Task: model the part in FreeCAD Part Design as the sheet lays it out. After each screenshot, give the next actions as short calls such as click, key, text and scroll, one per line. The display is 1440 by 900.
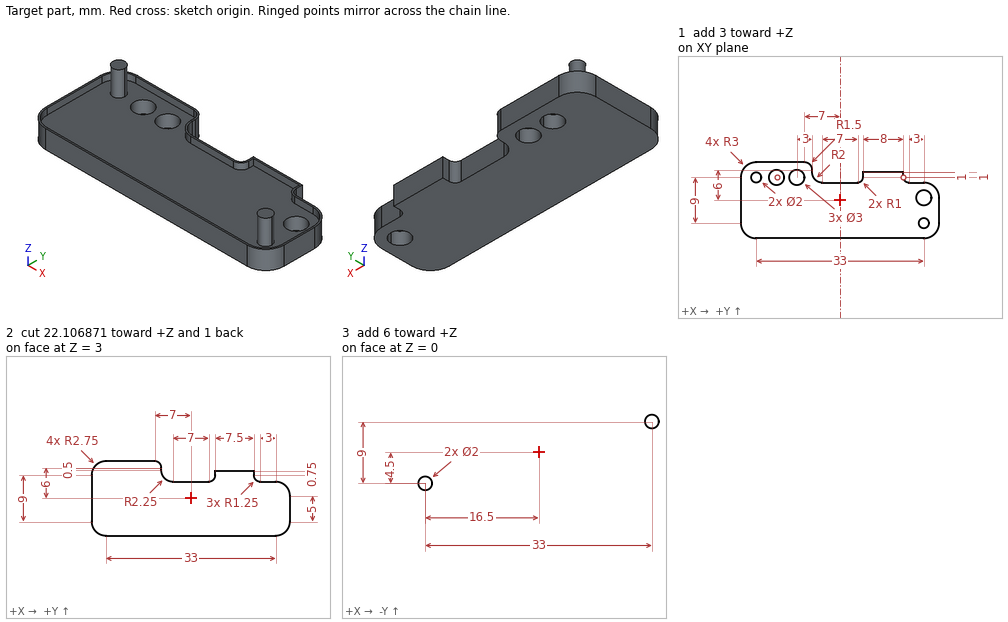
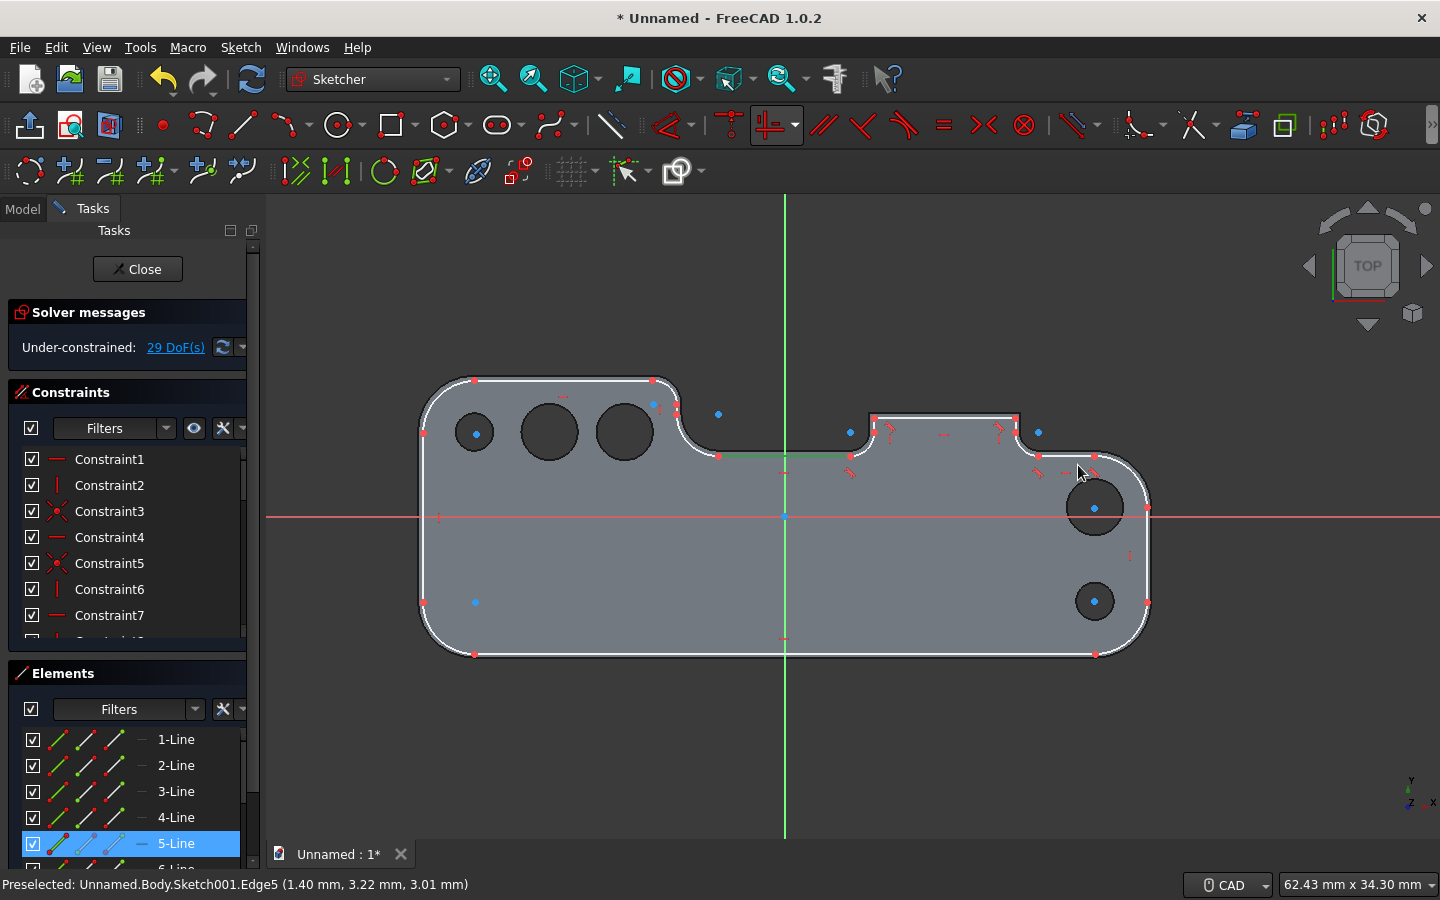
click(681, 433)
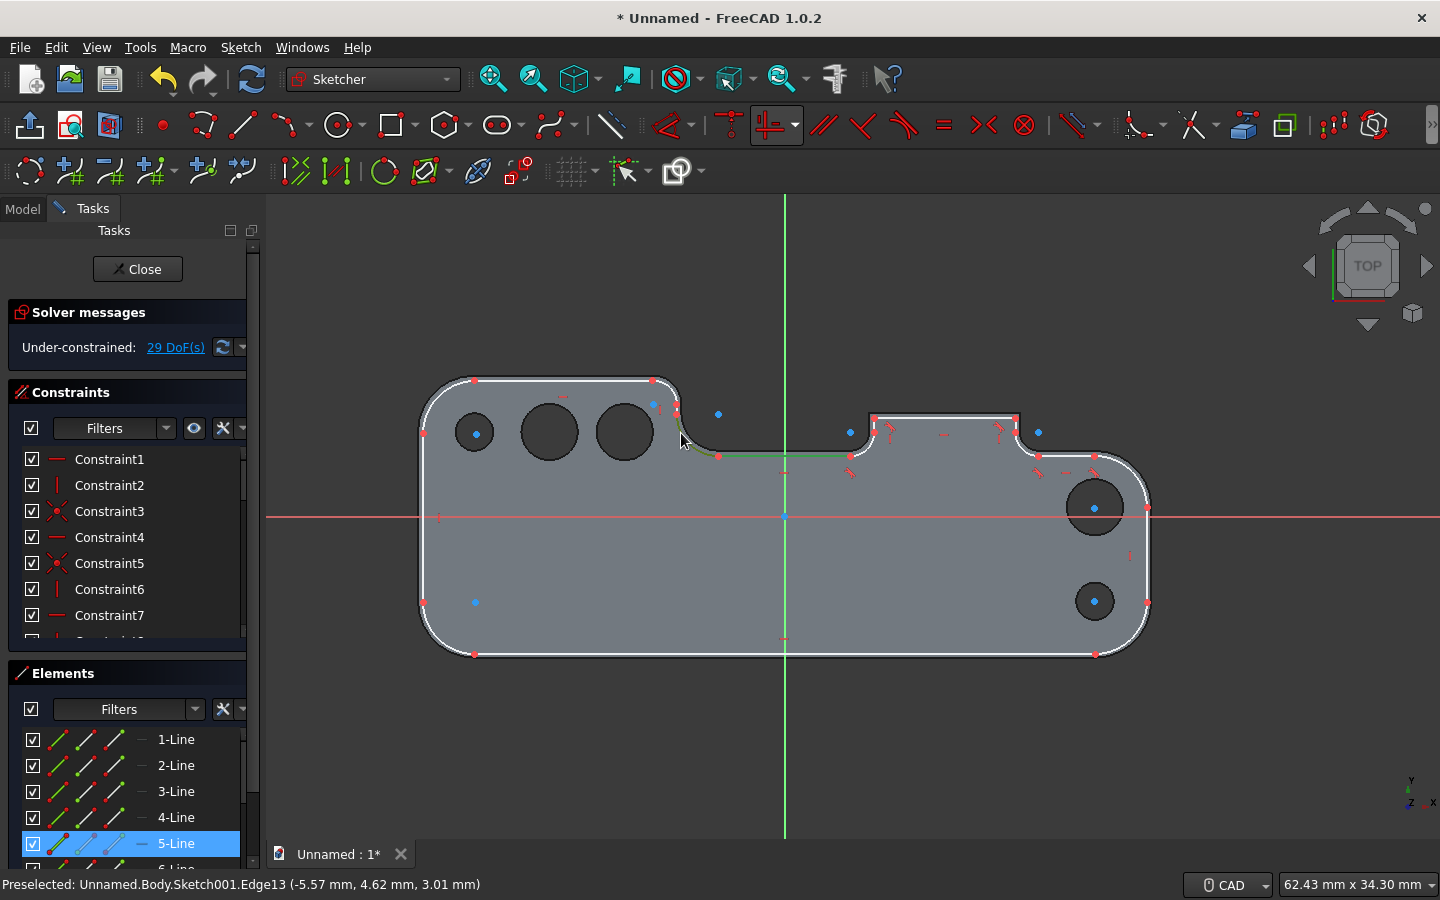
click(904, 126)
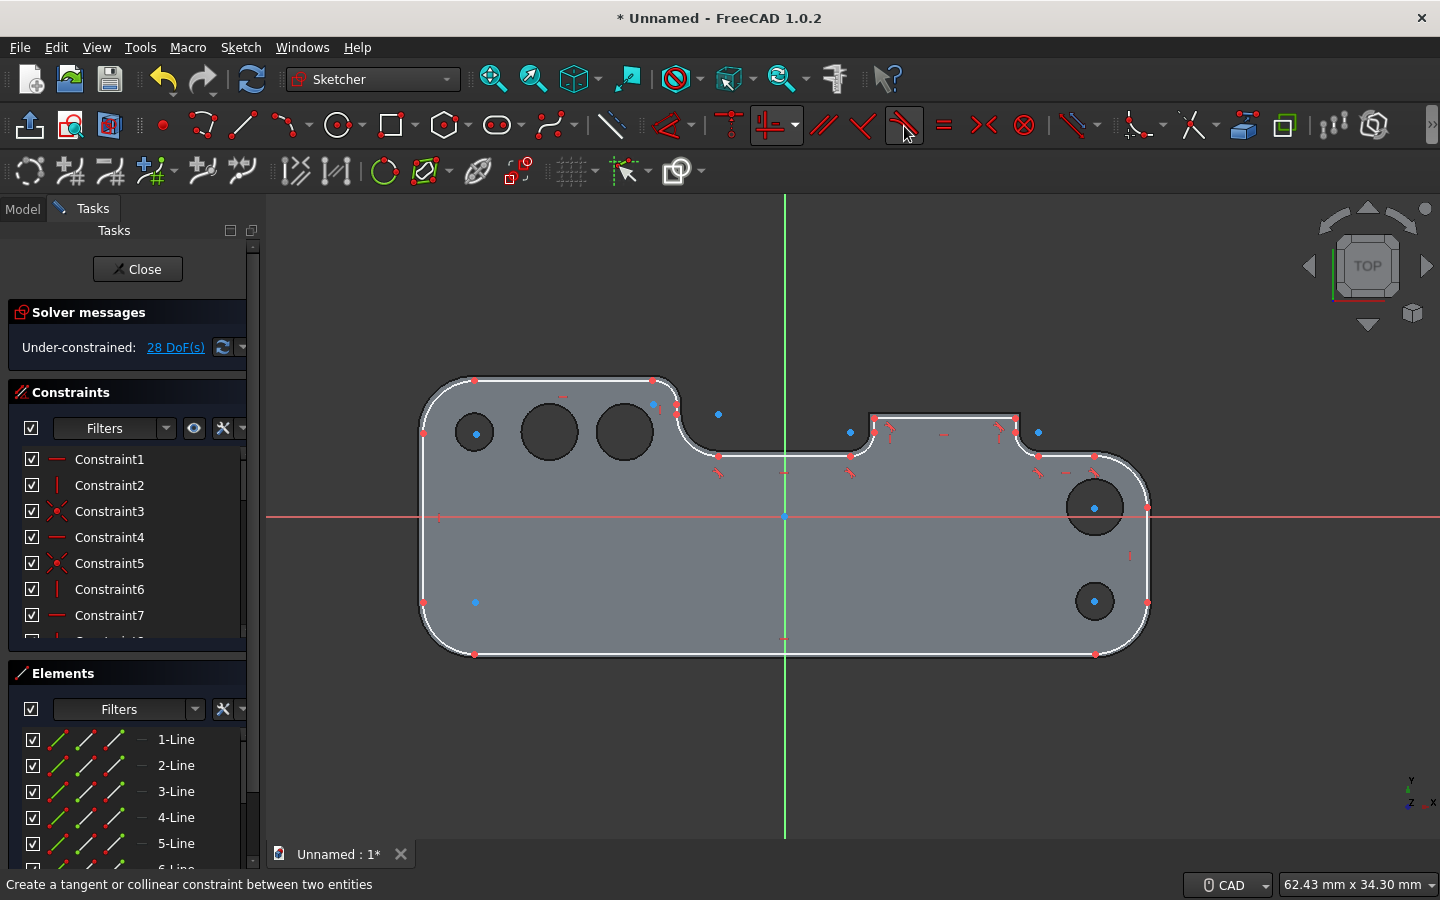
scroll(677, 409, up, 6)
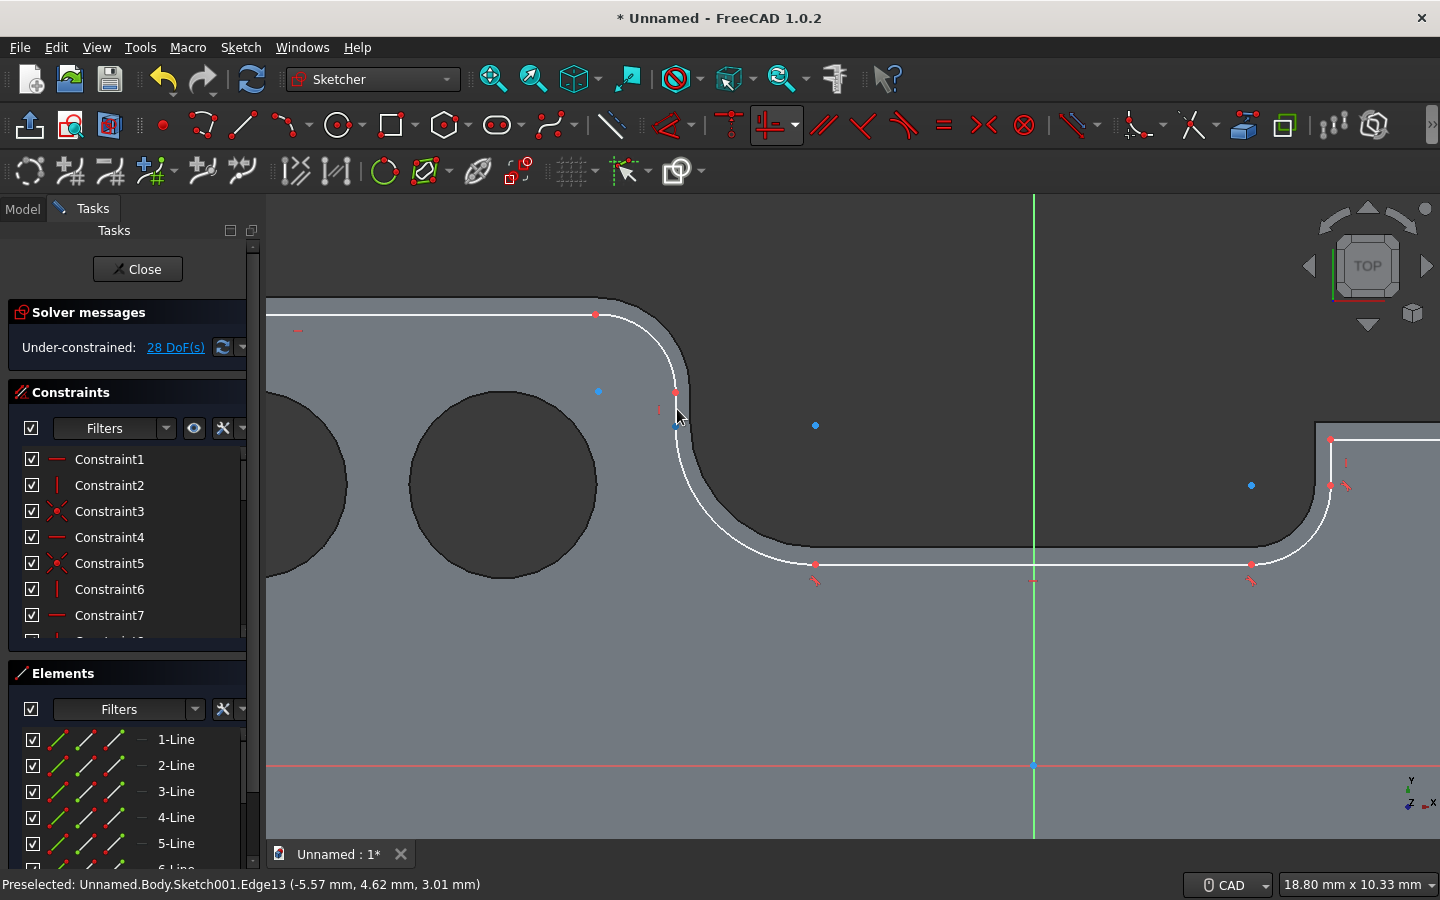
click(676, 410)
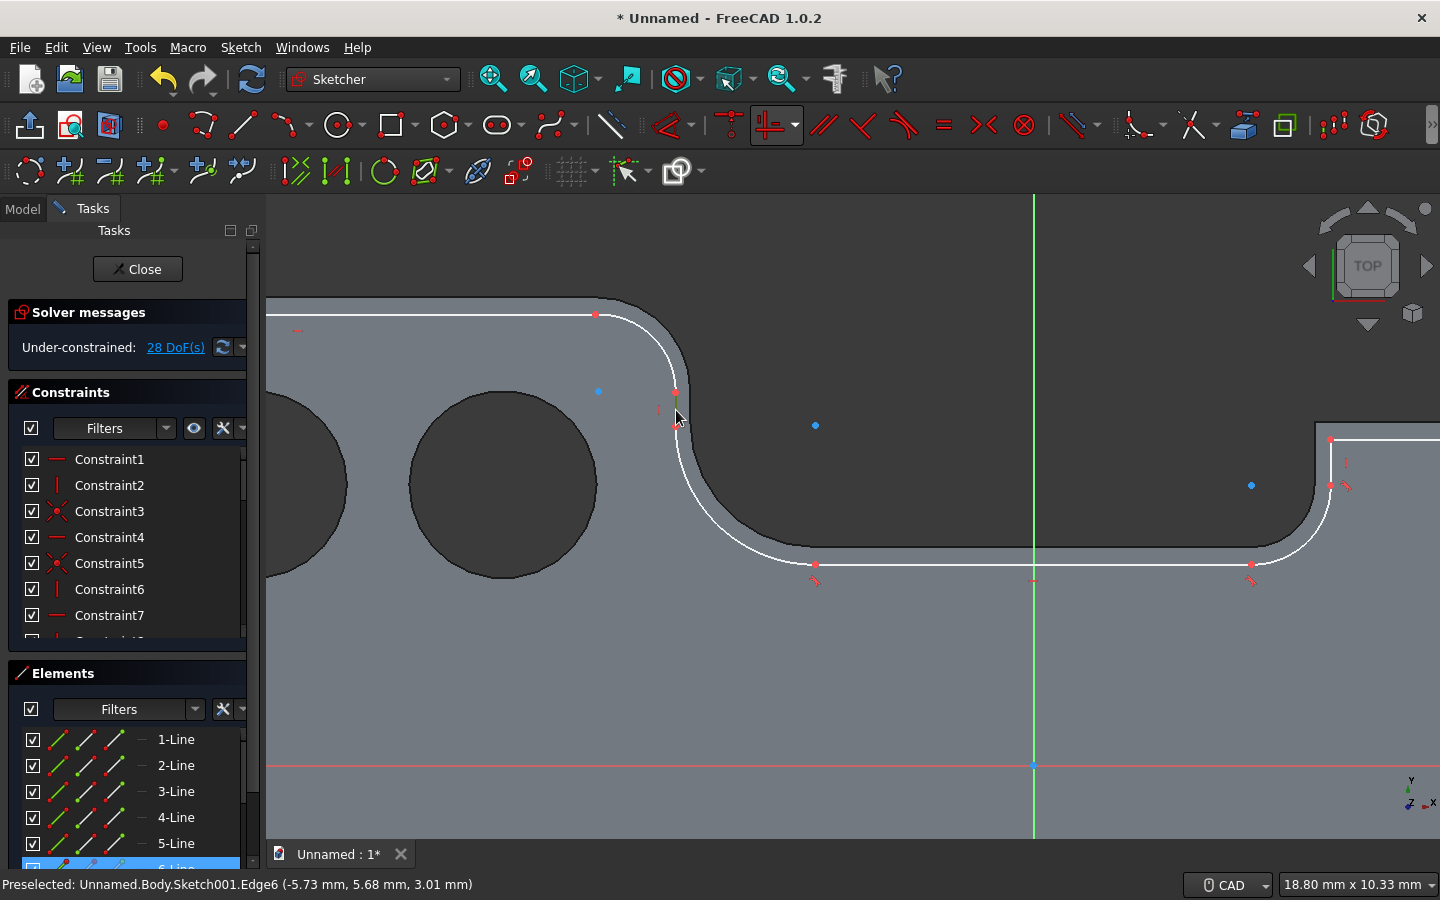
scroll(677, 409, down, 6)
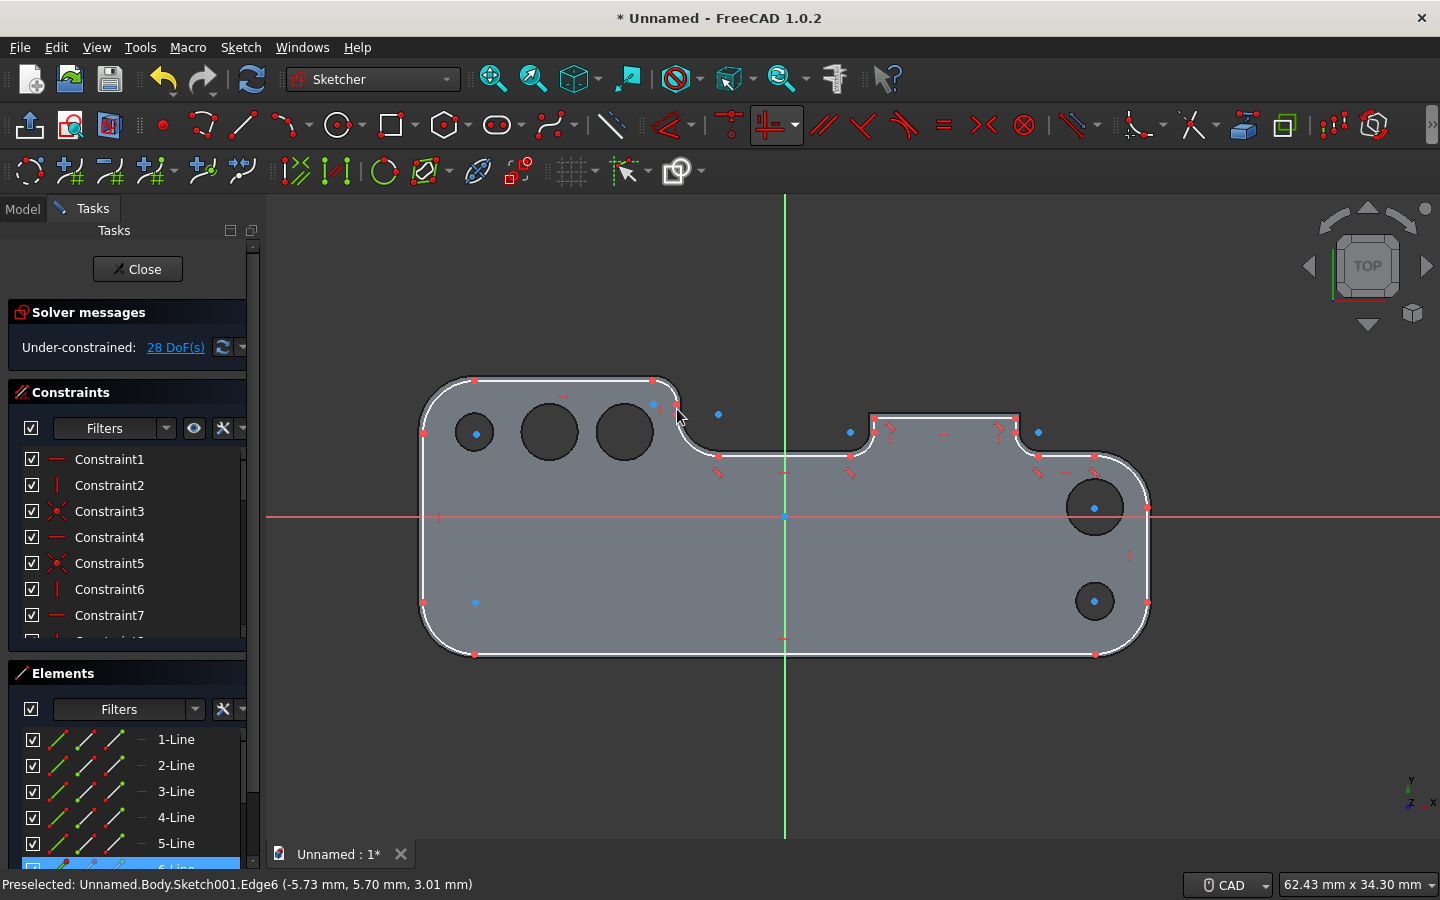
click(682, 433)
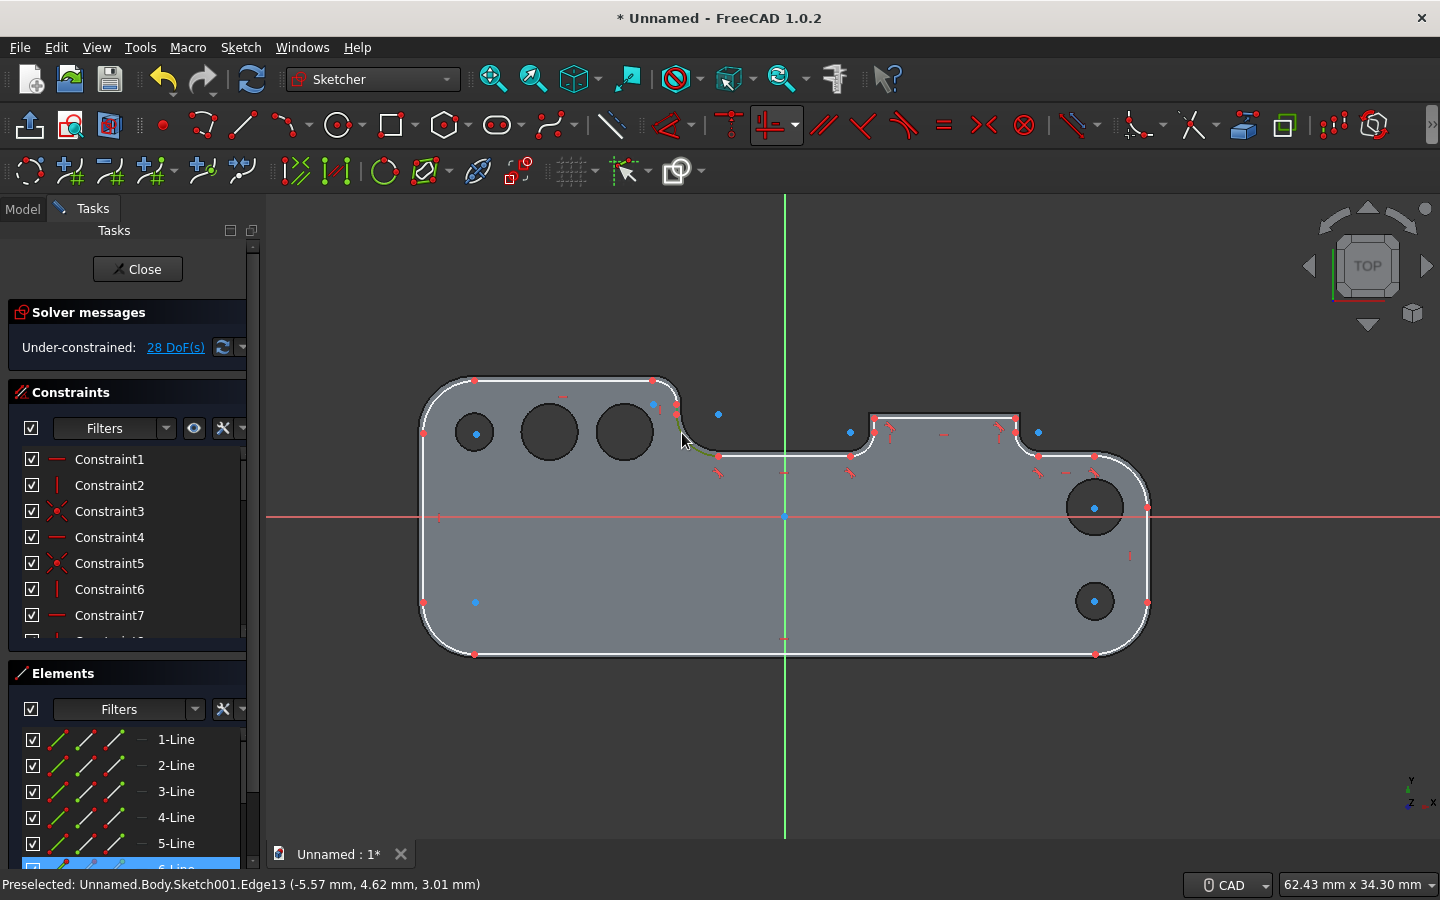
key(t)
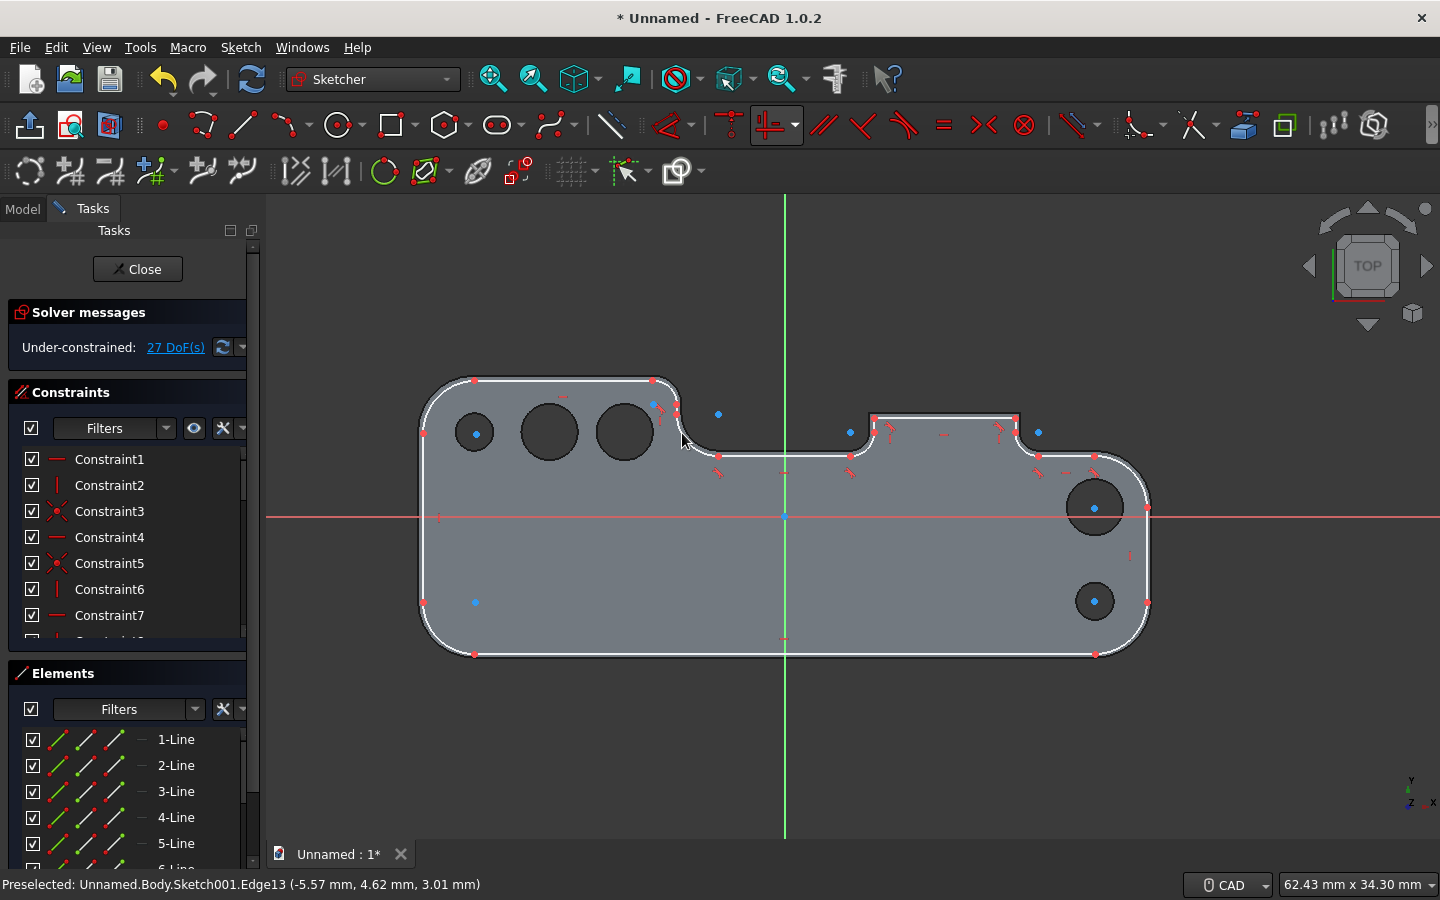
scroll(677, 409, up, 6)